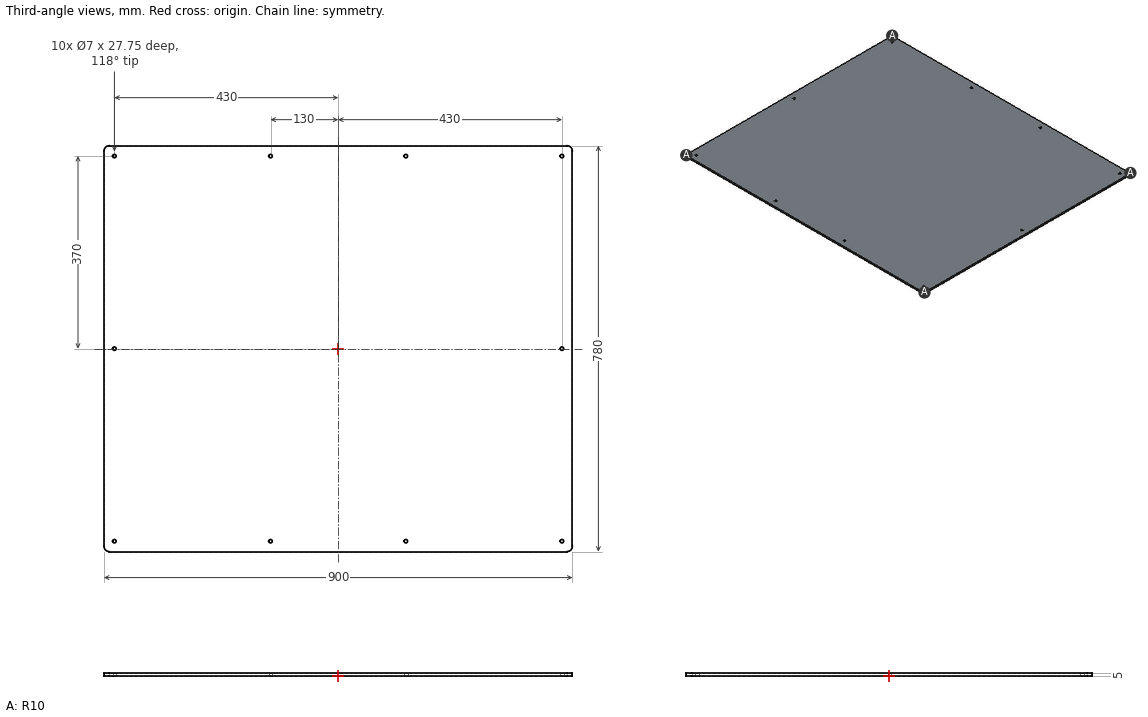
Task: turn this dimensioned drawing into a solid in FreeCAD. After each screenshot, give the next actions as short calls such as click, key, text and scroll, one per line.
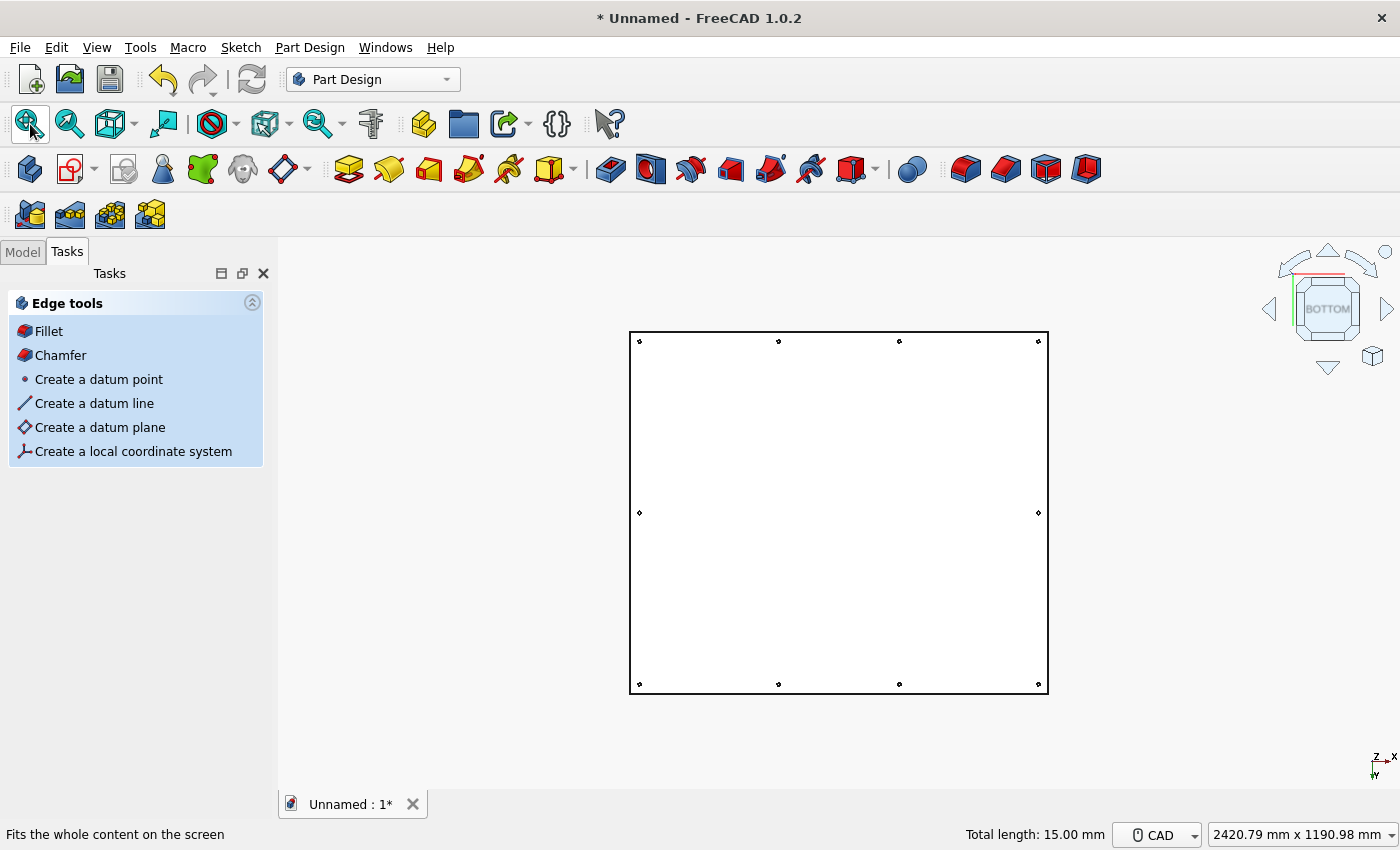
scroll(630, 693, up, 15)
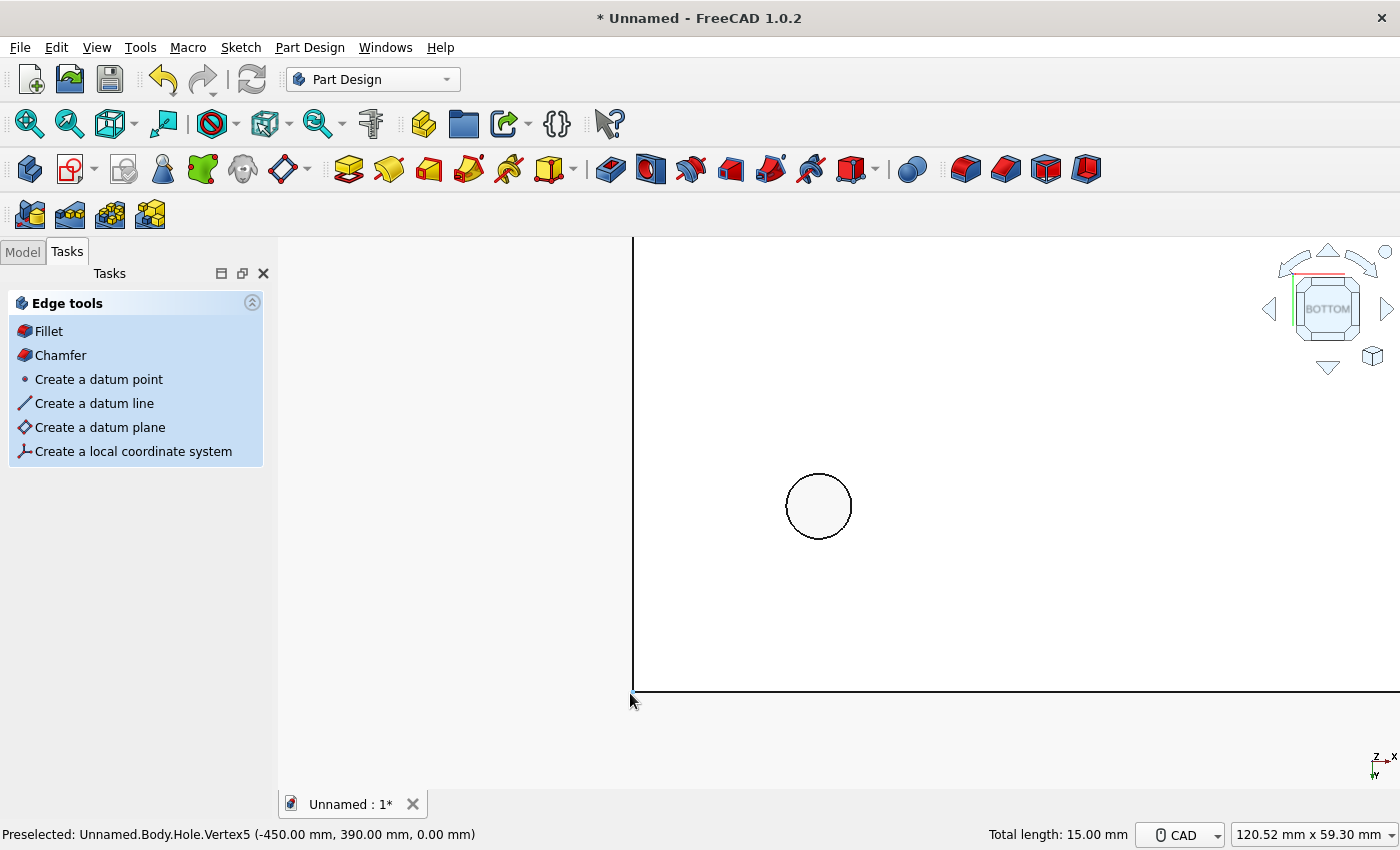
click(30, 124)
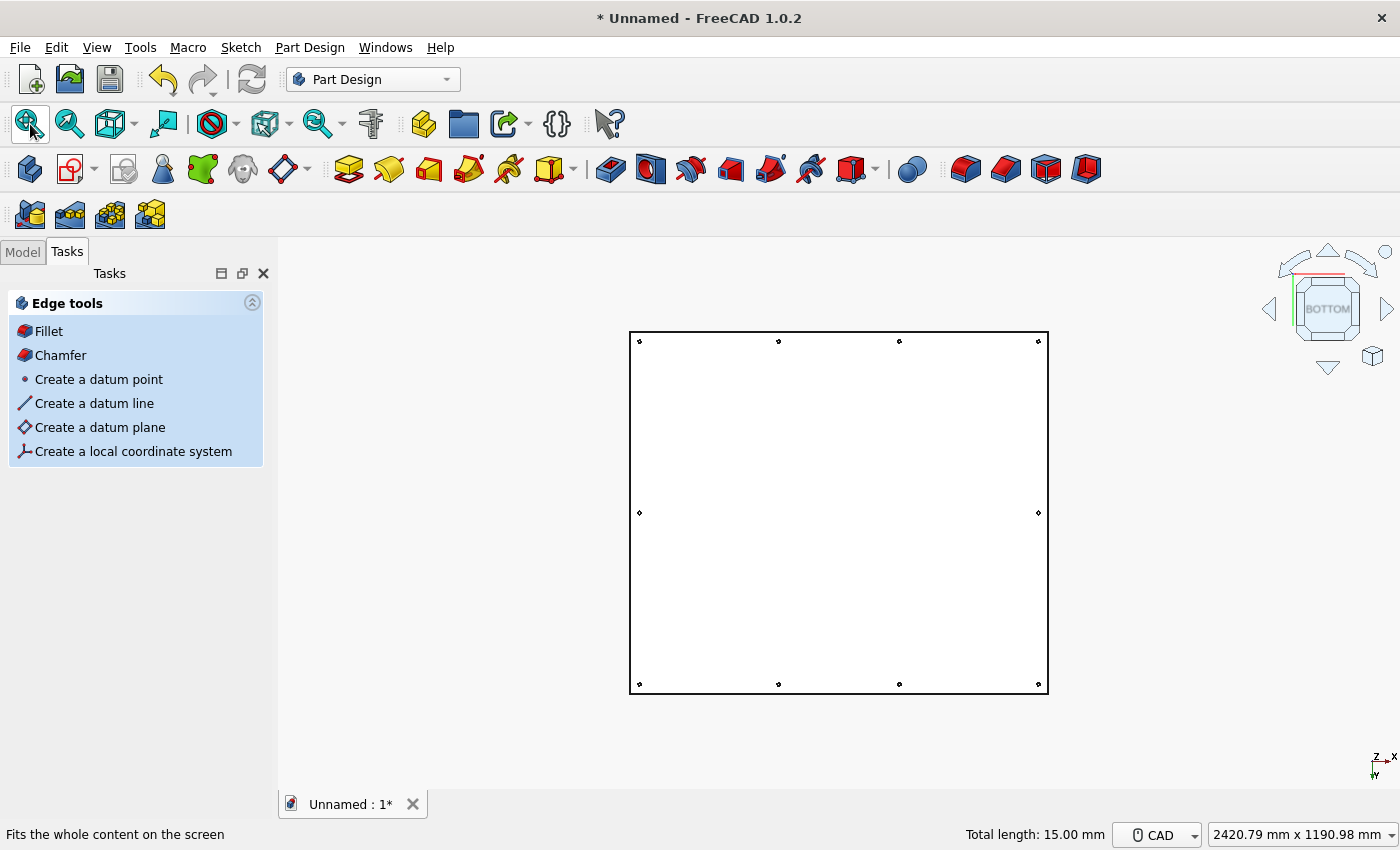
key(4)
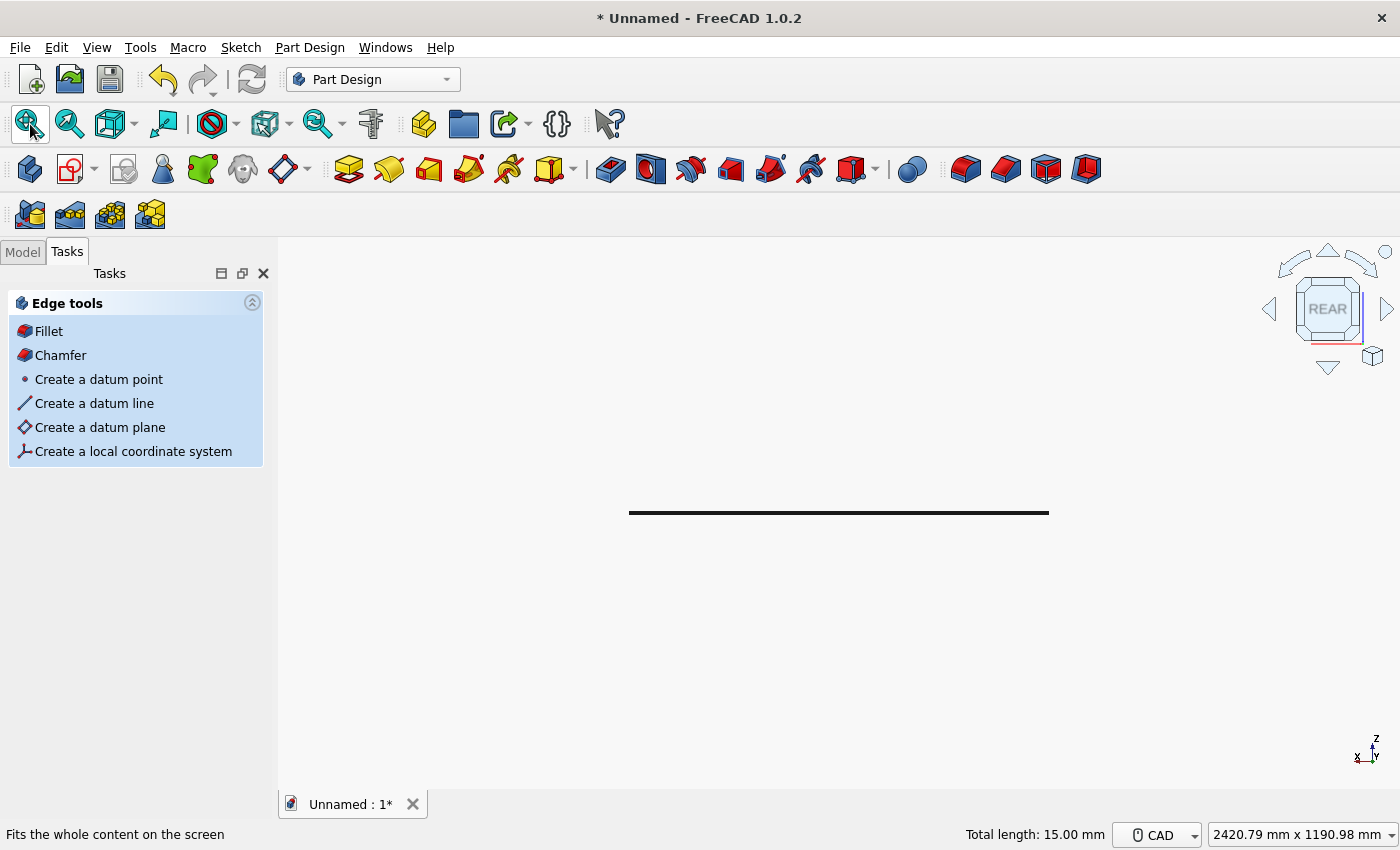
key(v)
key(f)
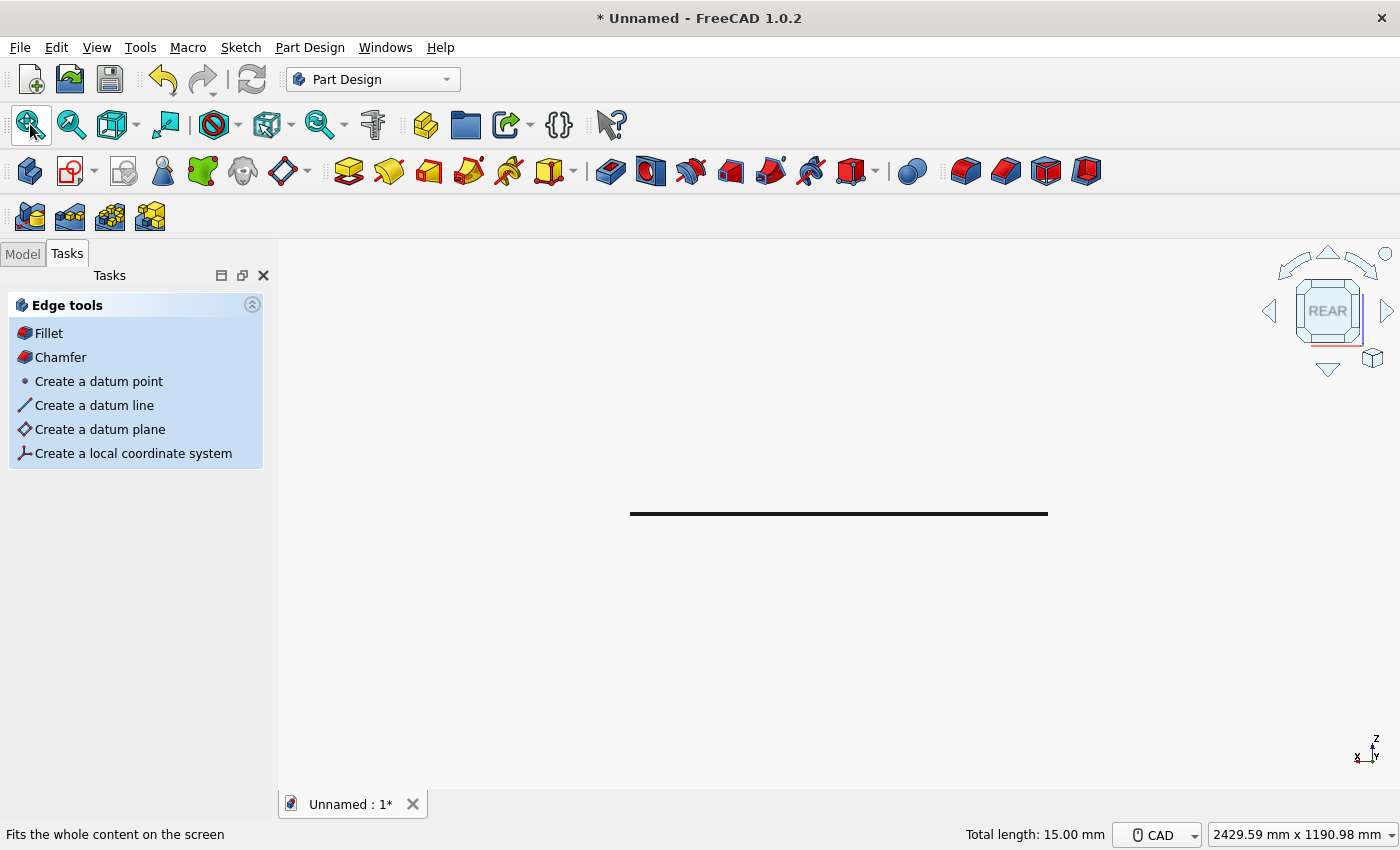
scroll(1047, 513, up, 15)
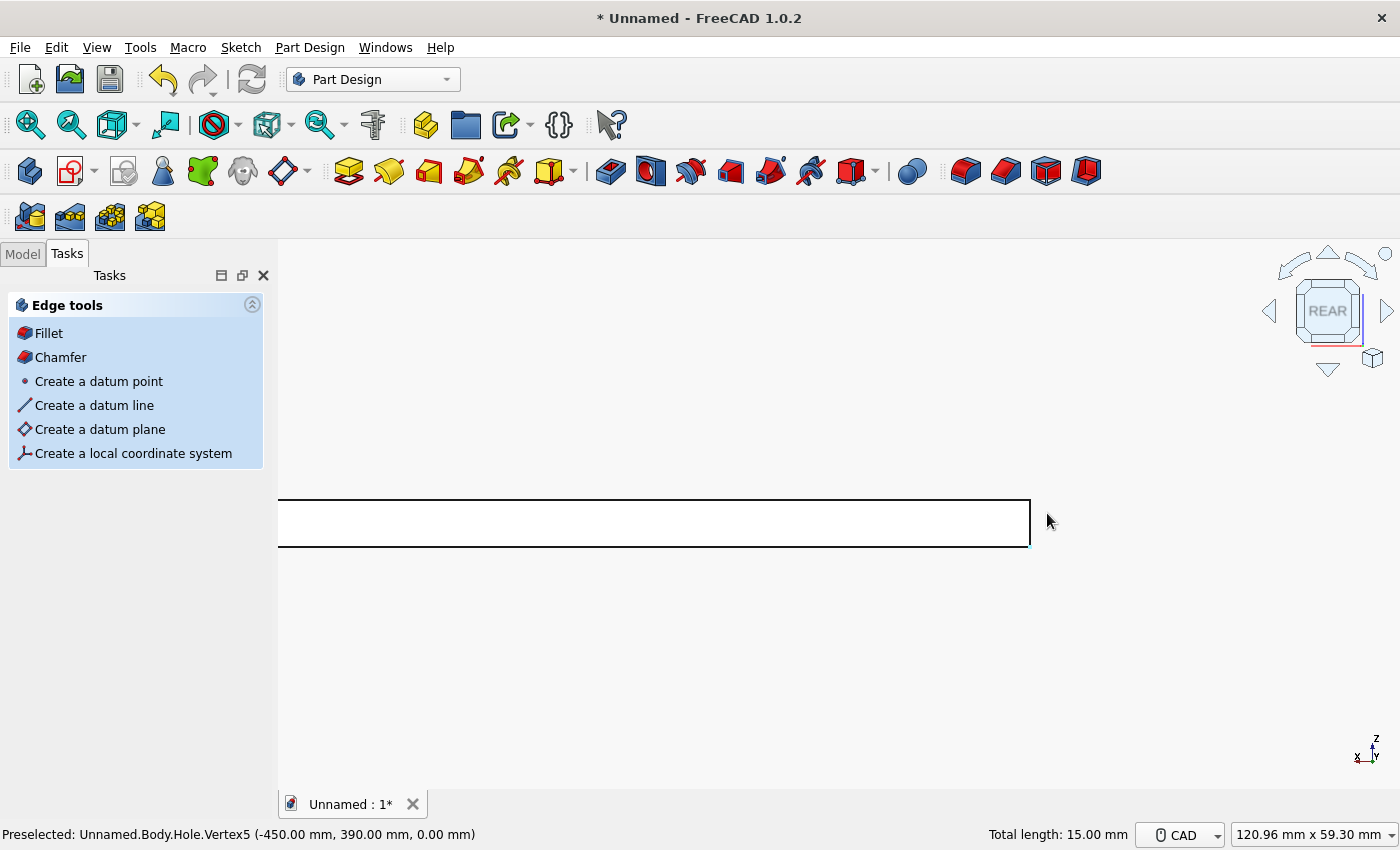
click(1030, 523, ctrl)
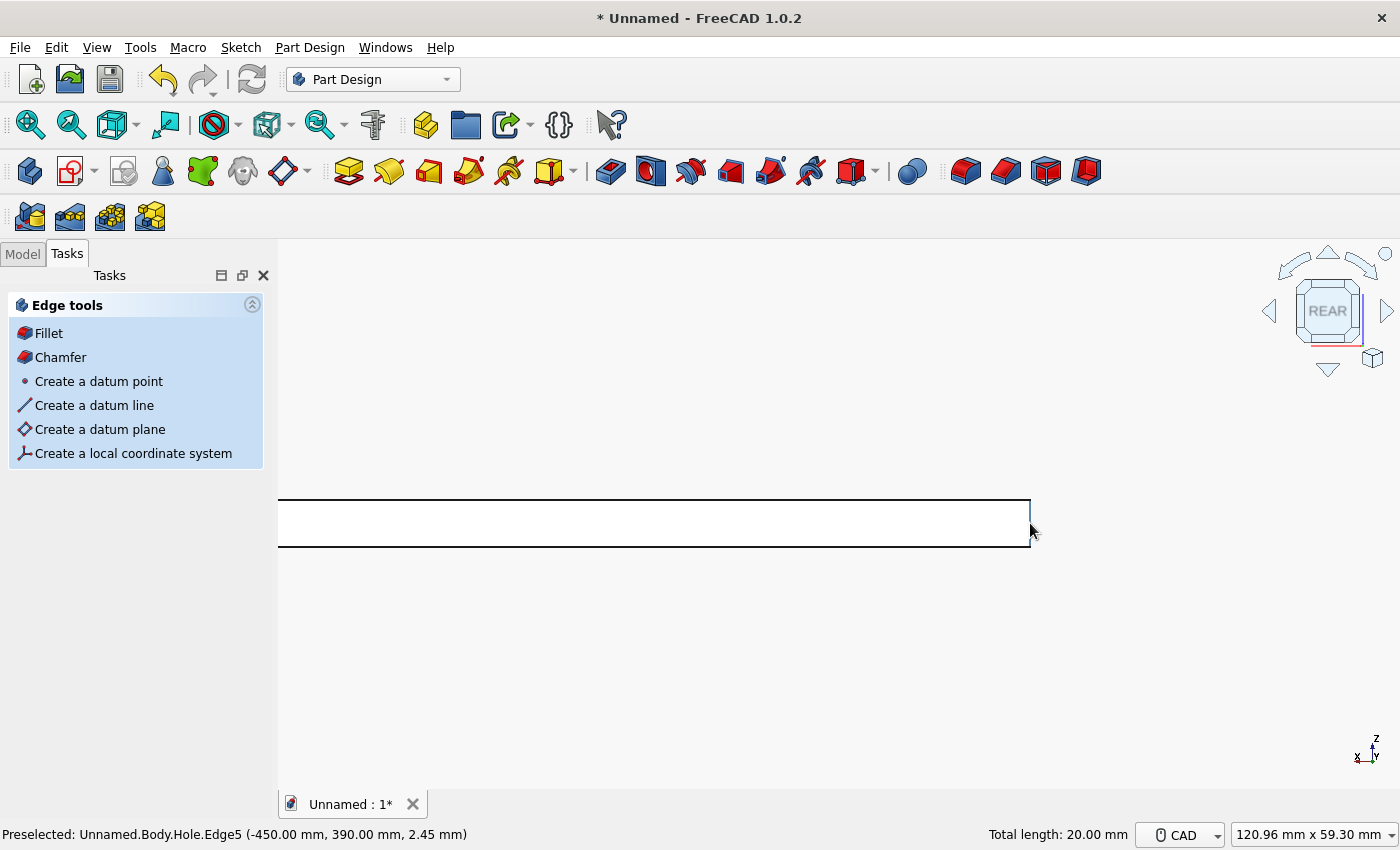
click(966, 172)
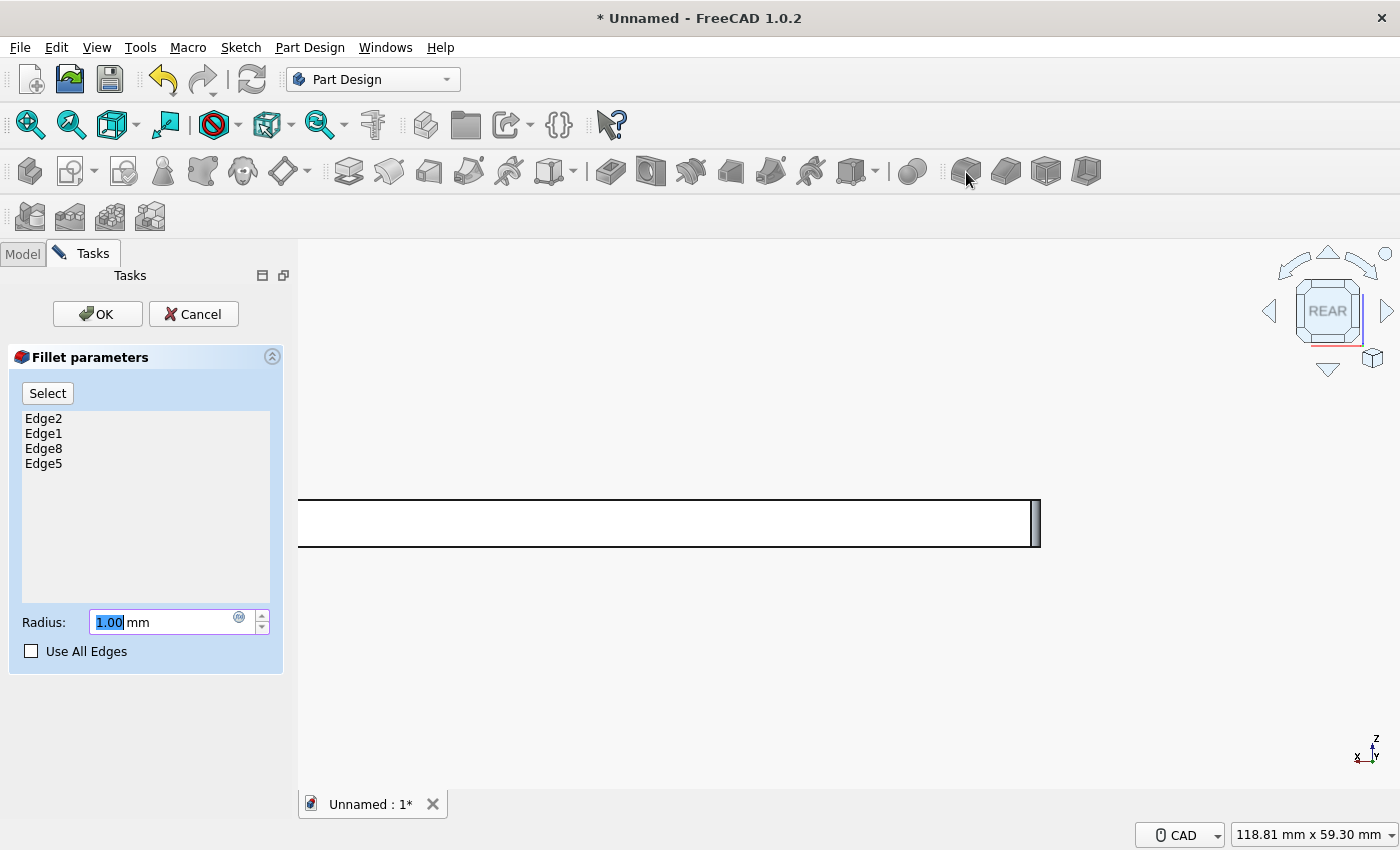
text(10)
key(Tab)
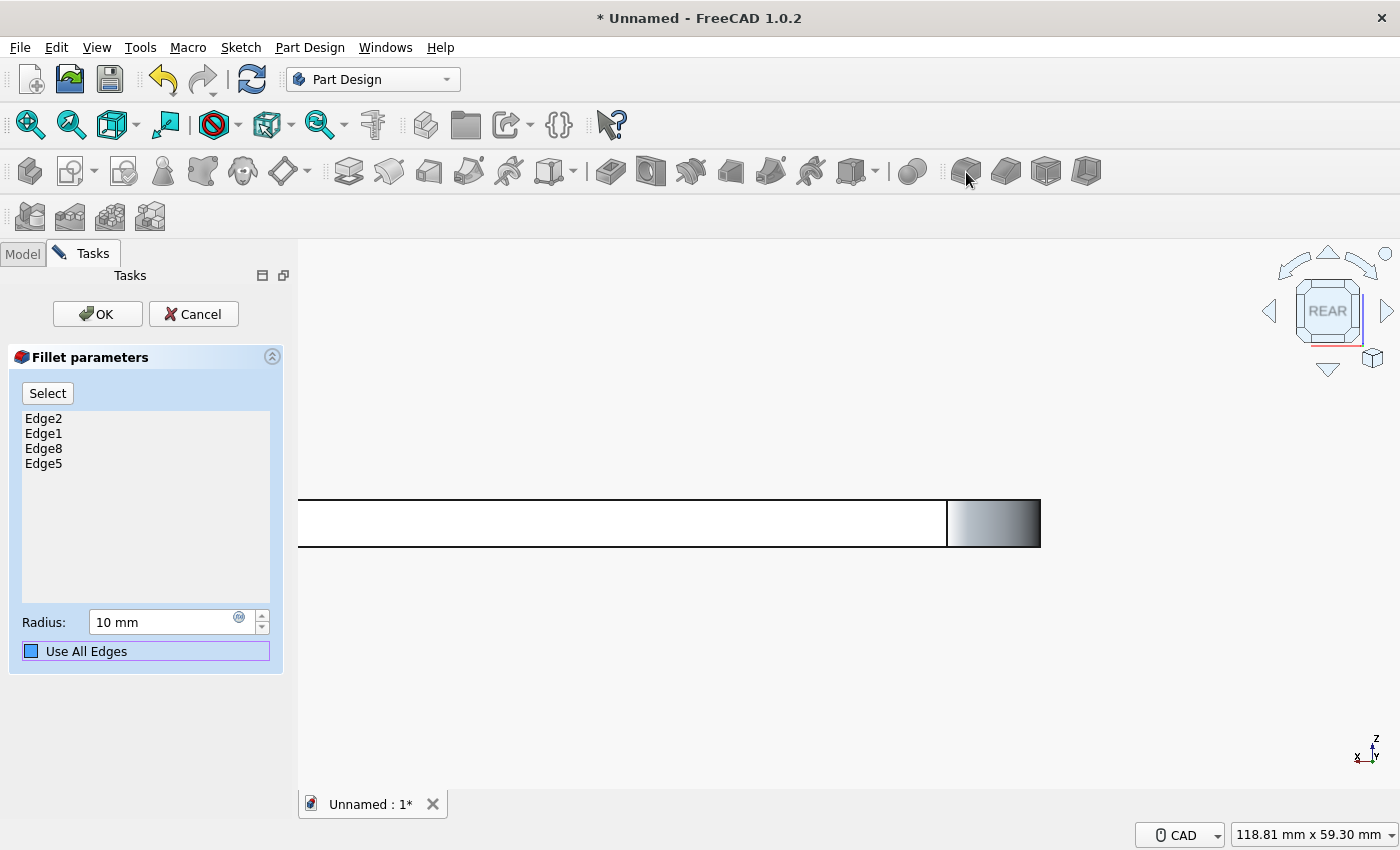
click(98, 314)